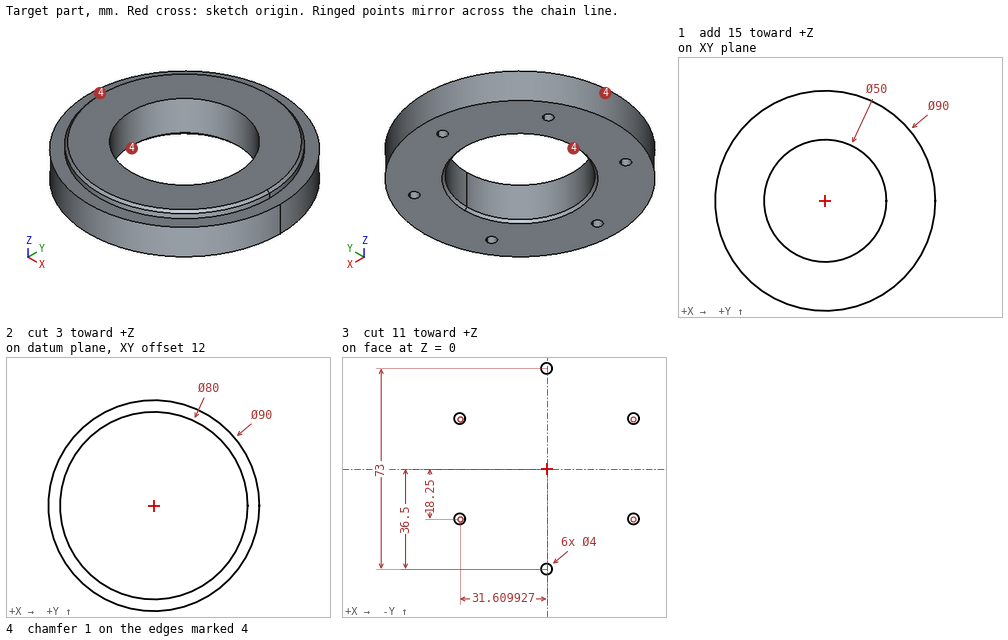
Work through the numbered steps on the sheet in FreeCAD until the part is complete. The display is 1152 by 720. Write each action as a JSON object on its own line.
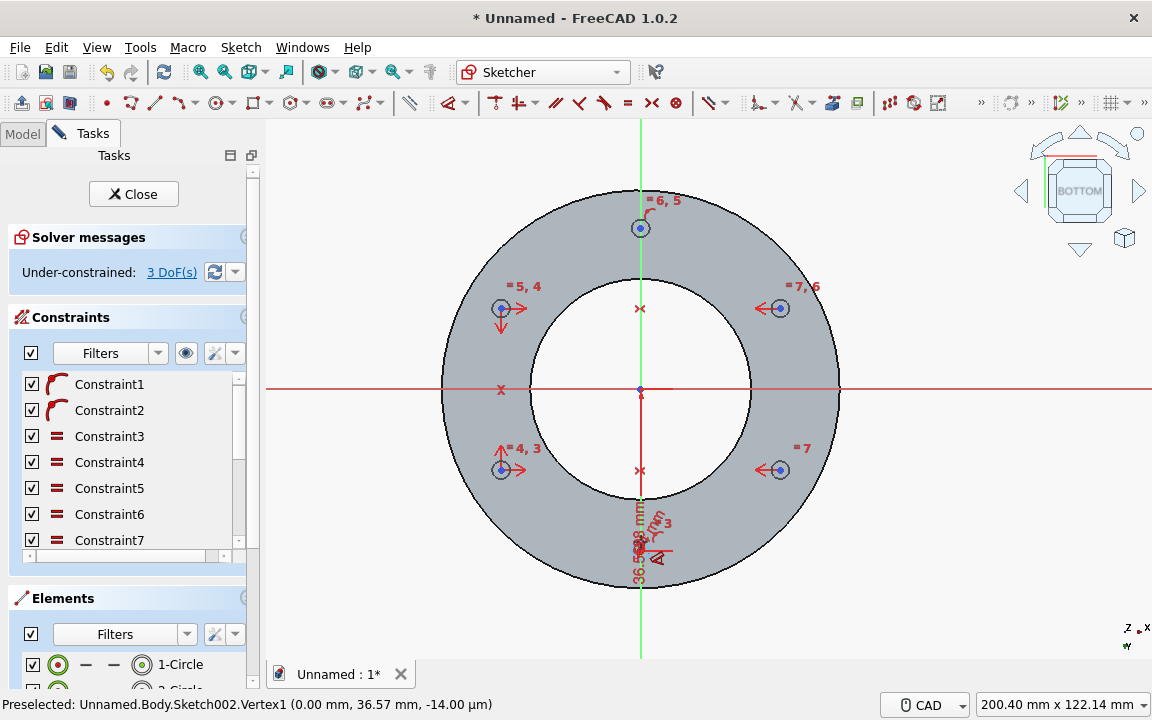
{"action": "left_click", "coordinate": [641, 228]}
{"action": "left_click", "coordinate": [675, 315]}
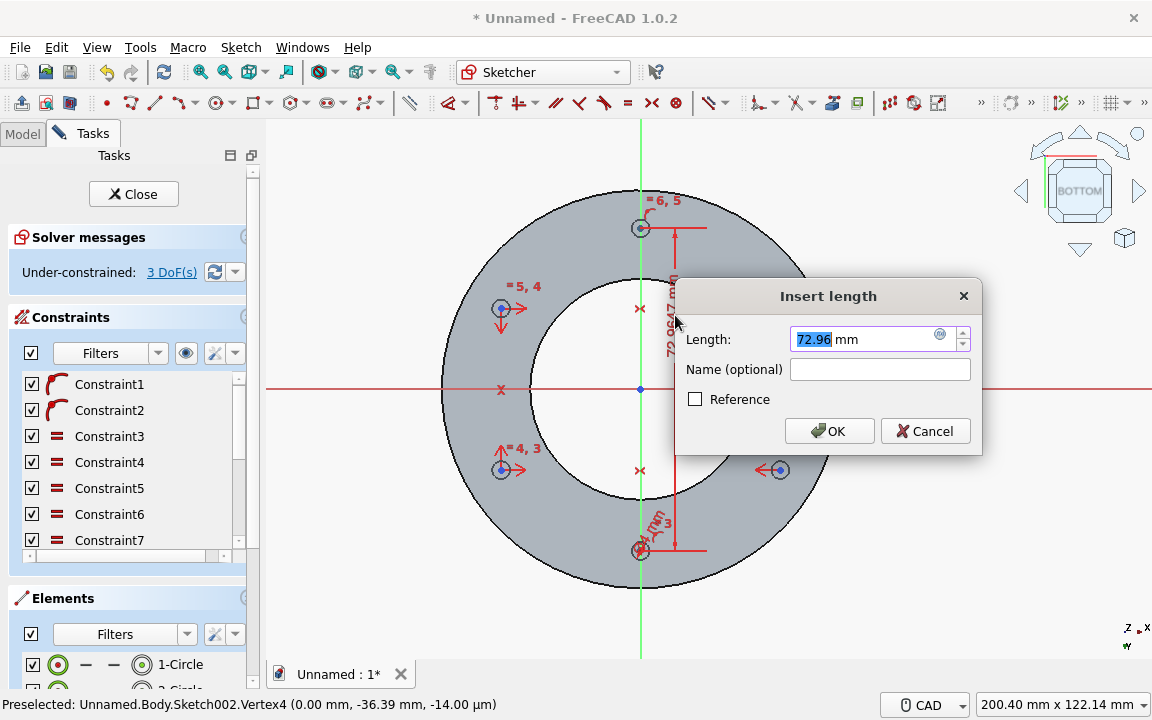
{"action": "type", "text": "73"}
{"action": "key", "text": "Return"}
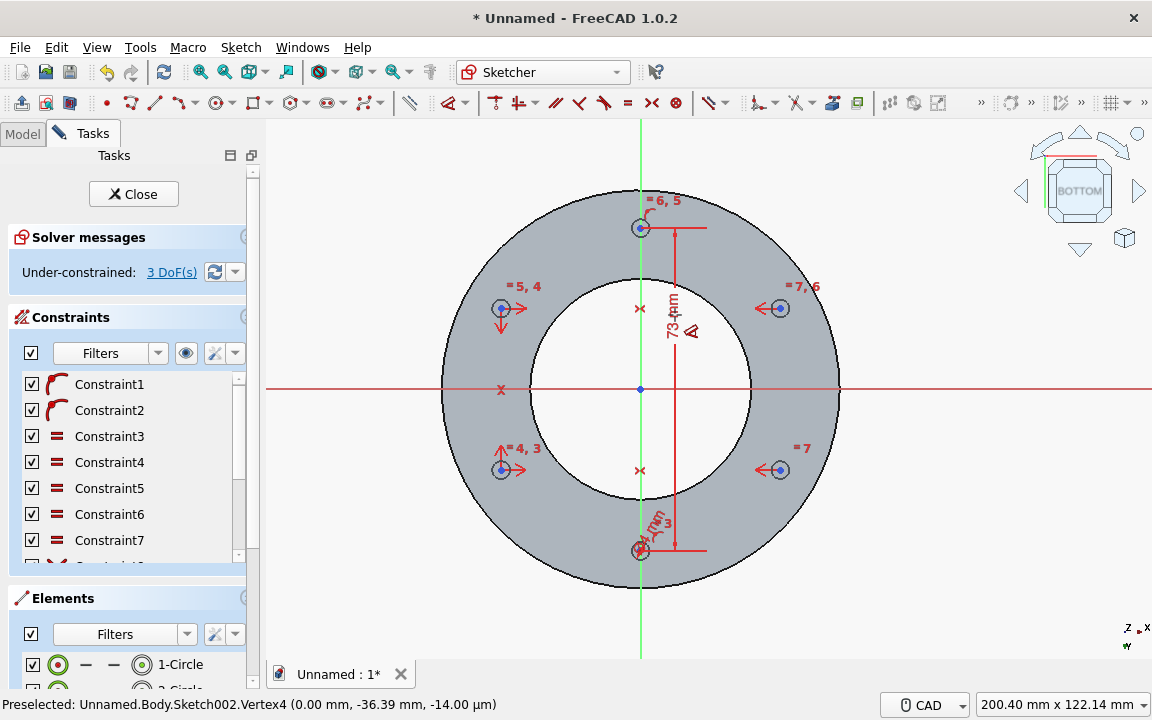
{"action": "left_click", "coordinate": [641, 551]}
{"action": "left_click", "coordinate": [675, 470]}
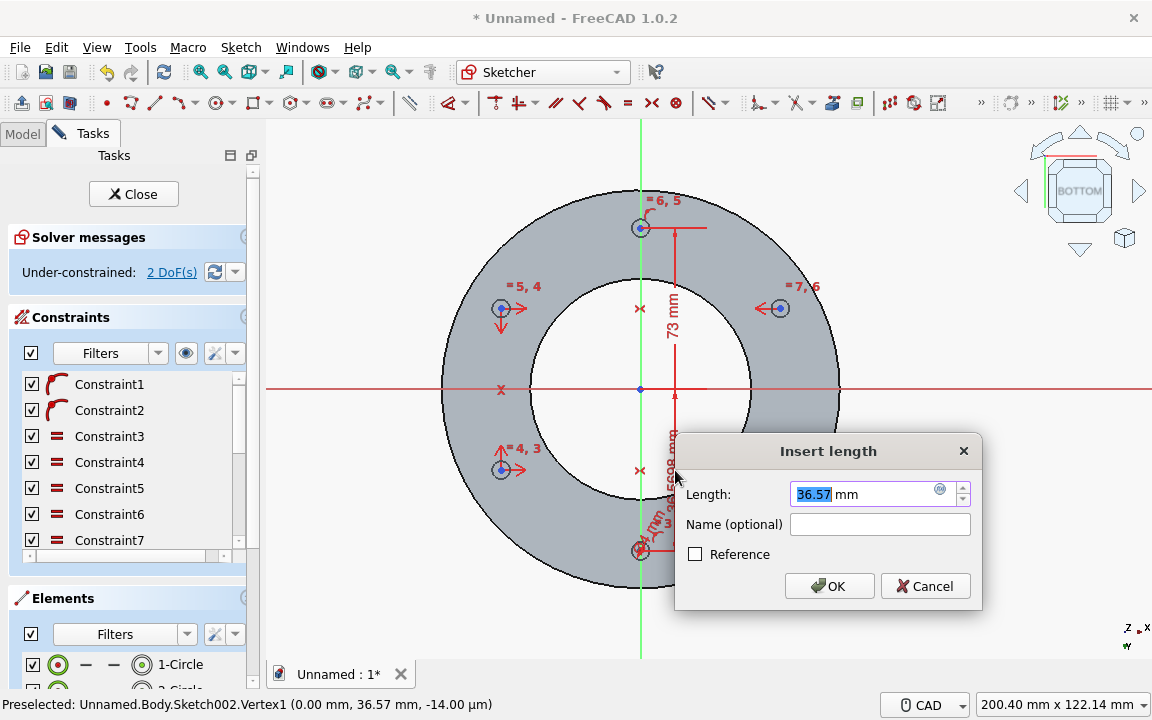
{"action": "type", "text": "36.5"}
{"action": "key", "text": "Return"}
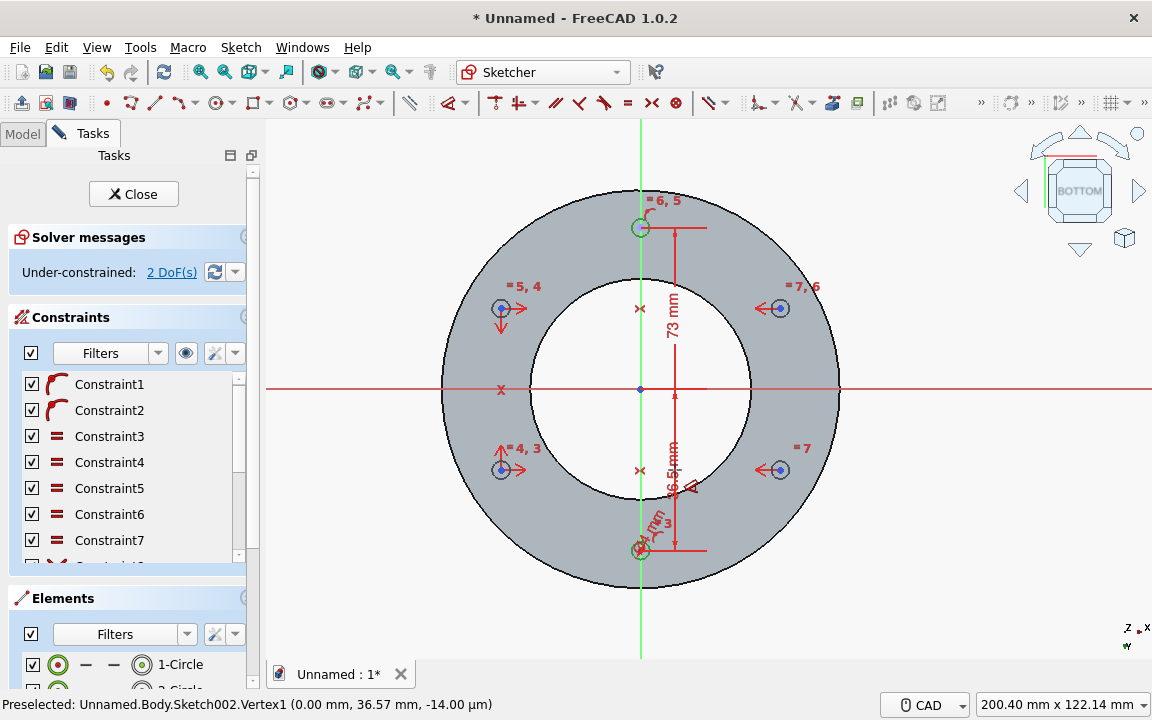
{"action": "left_click", "coordinate": [501, 470]}
{"action": "left_click", "coordinate": [467, 430]}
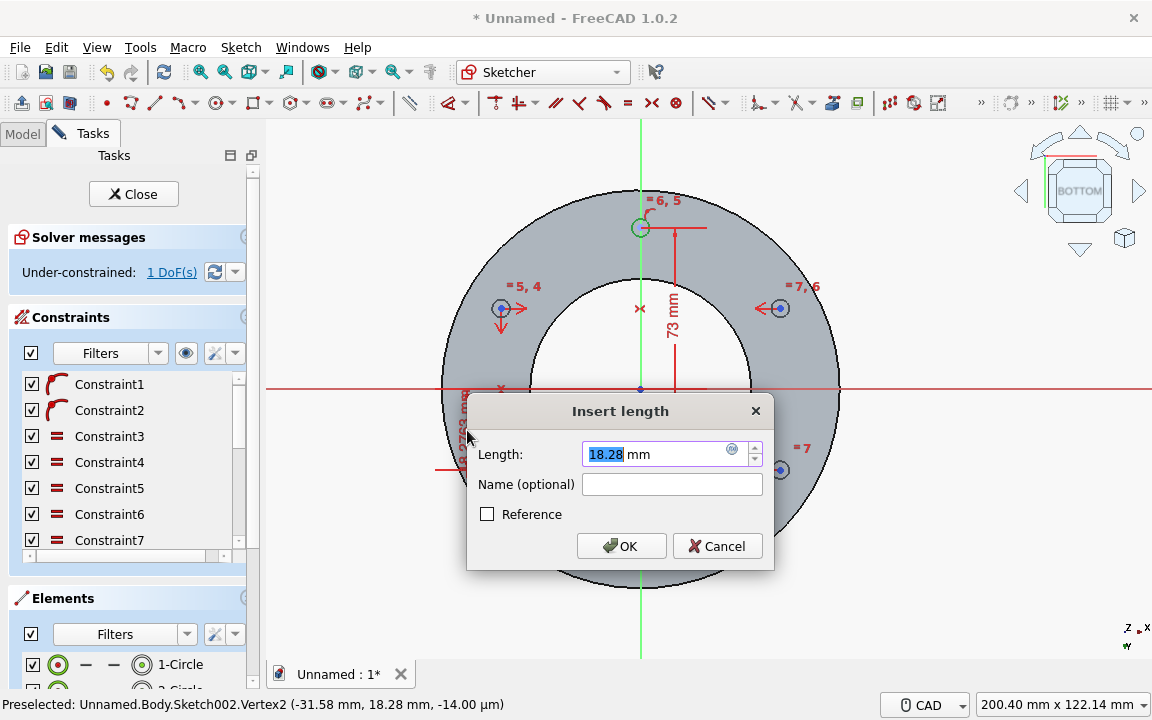
{"action": "type", "text": "18.25"}
{"action": "key", "text": "Return"}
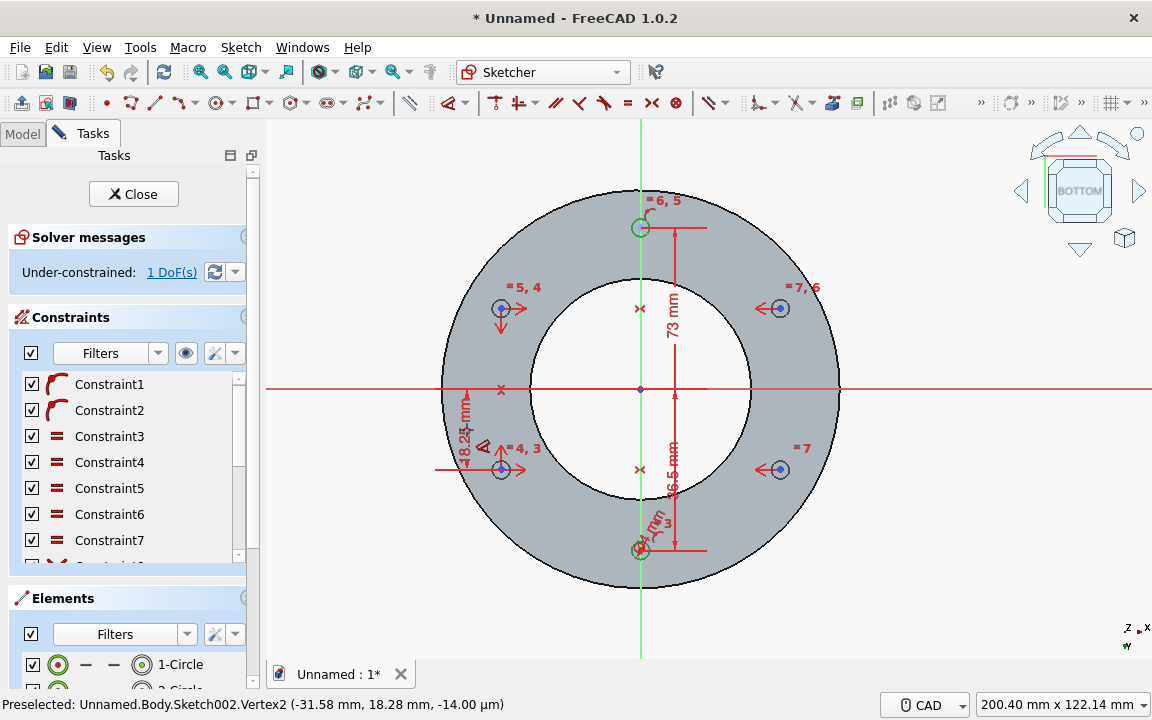
{"action": "left_click", "coordinate": [501, 470]}
{"action": "left_click", "coordinate": [571, 504]}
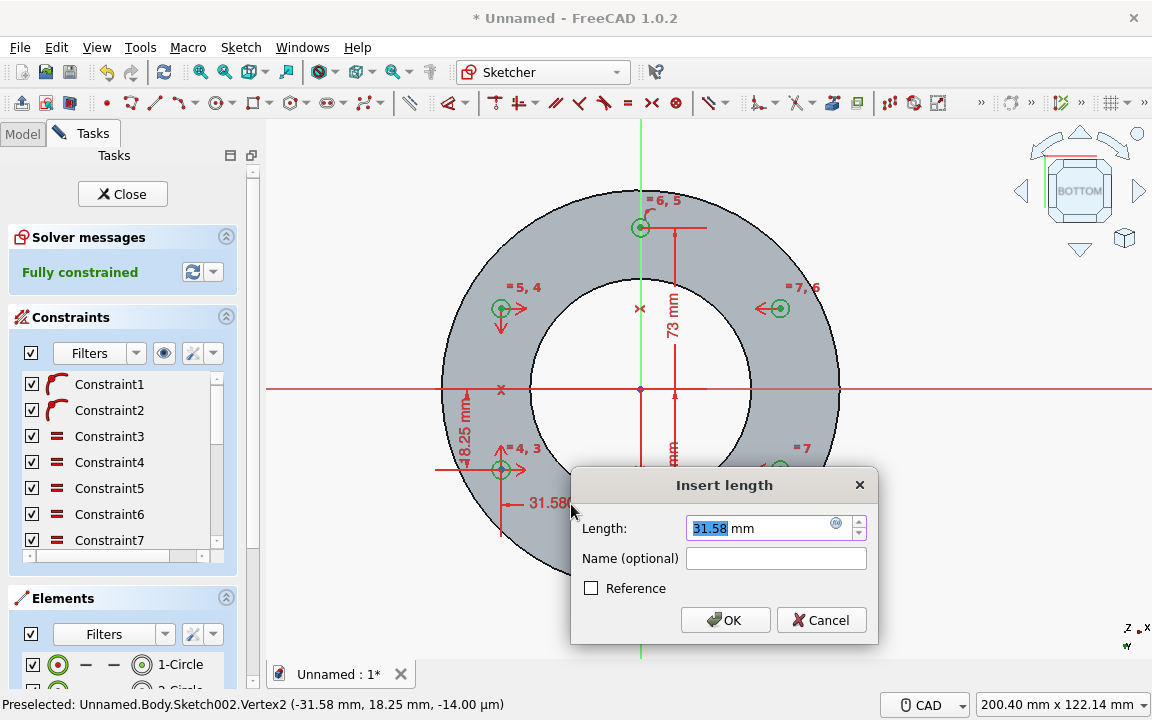
{"action": "type", "text": "31.609927"}
{"action": "key", "text": "Return"}
{"action": "key", "text": "Escape"}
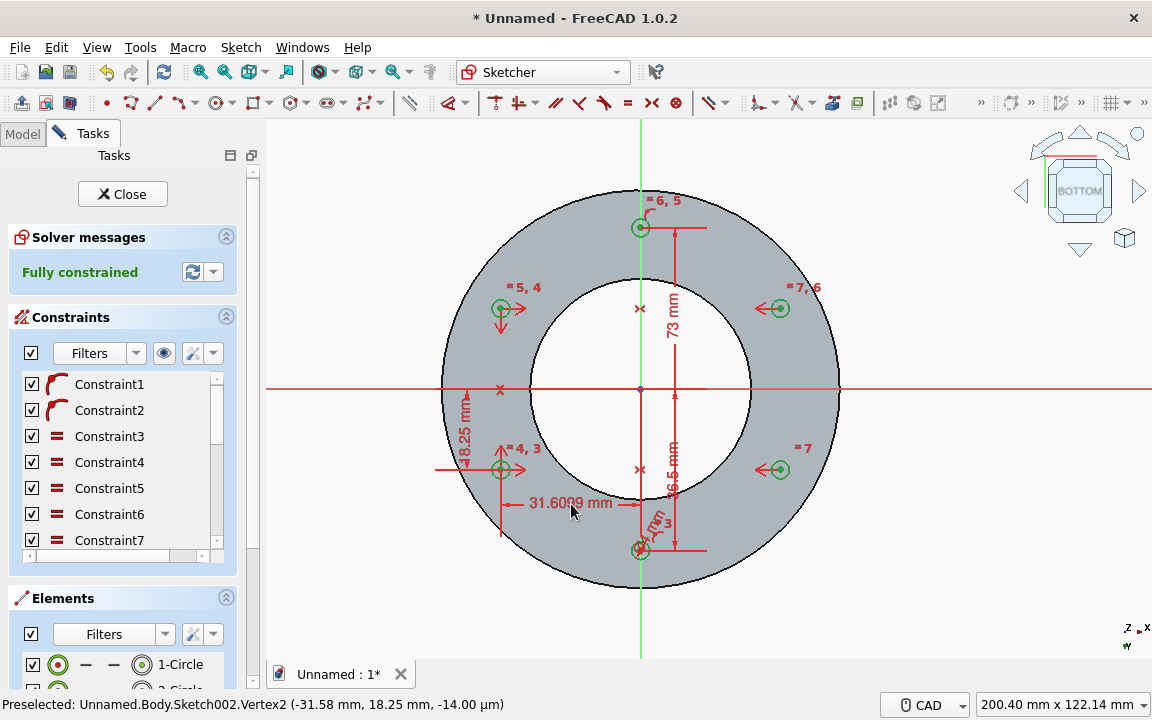
{"action": "left_click", "coordinate": [123, 194]}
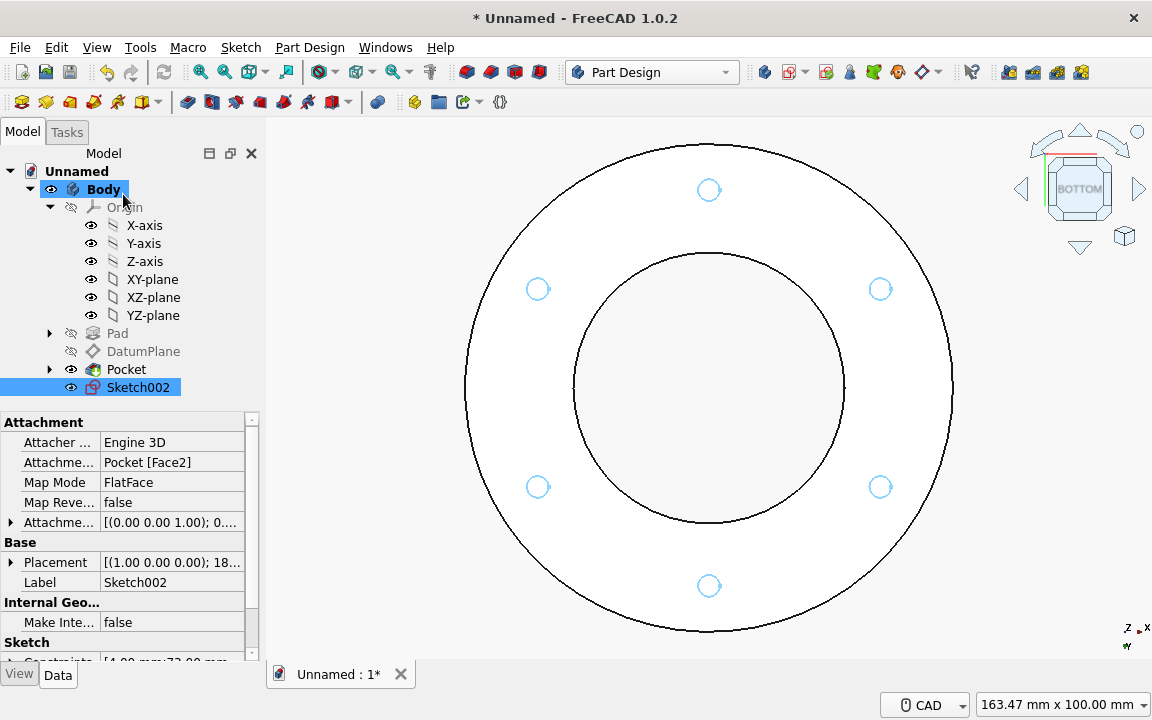
{"action": "left_click", "coordinate": [188, 102]}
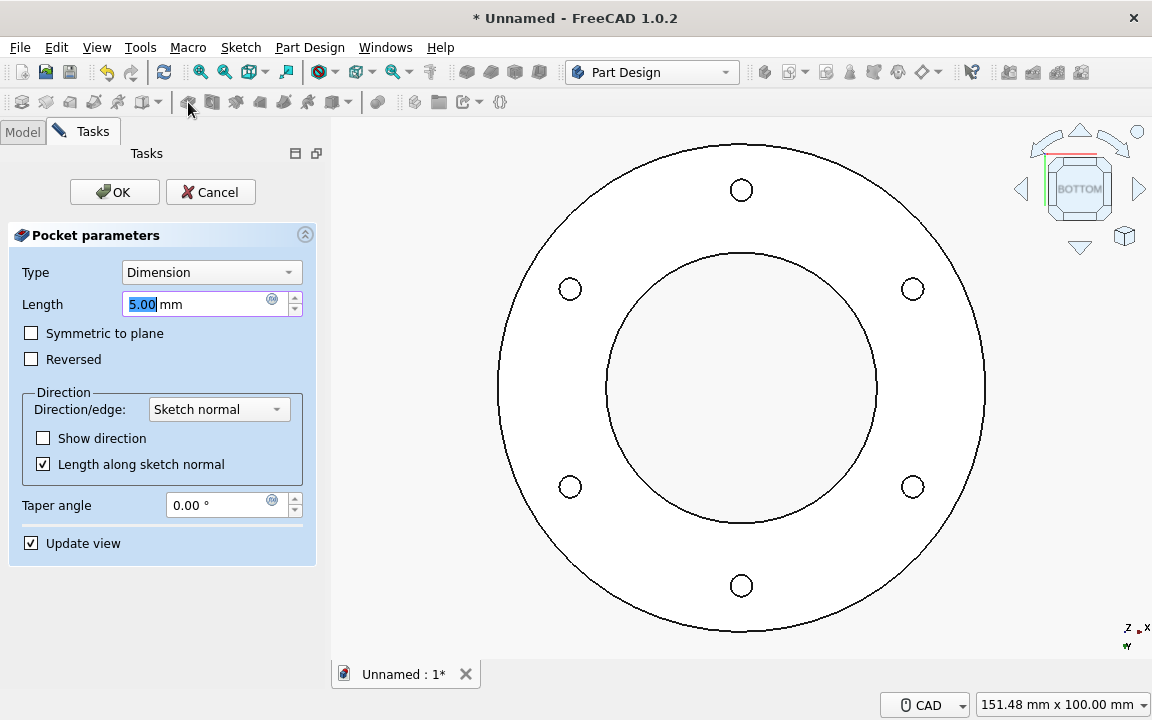
{"action": "type", "text": "11"}
{"action": "key", "text": "Tab"}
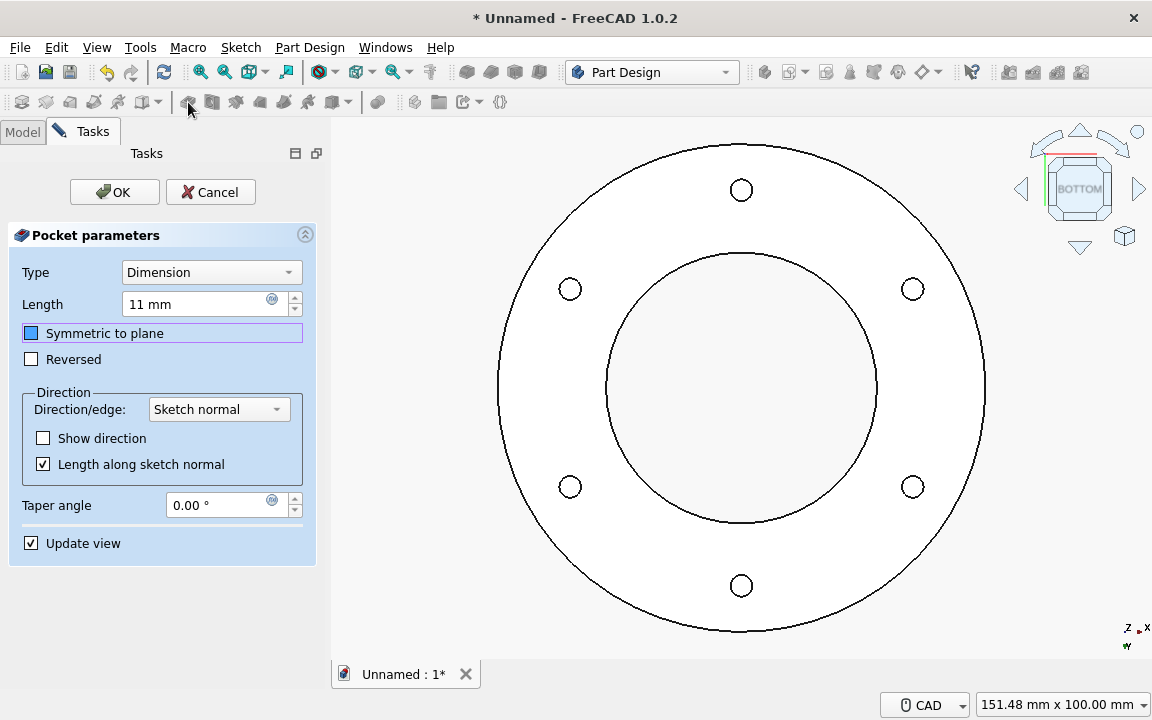
{"action": "left_click", "coordinate": [115, 192]}